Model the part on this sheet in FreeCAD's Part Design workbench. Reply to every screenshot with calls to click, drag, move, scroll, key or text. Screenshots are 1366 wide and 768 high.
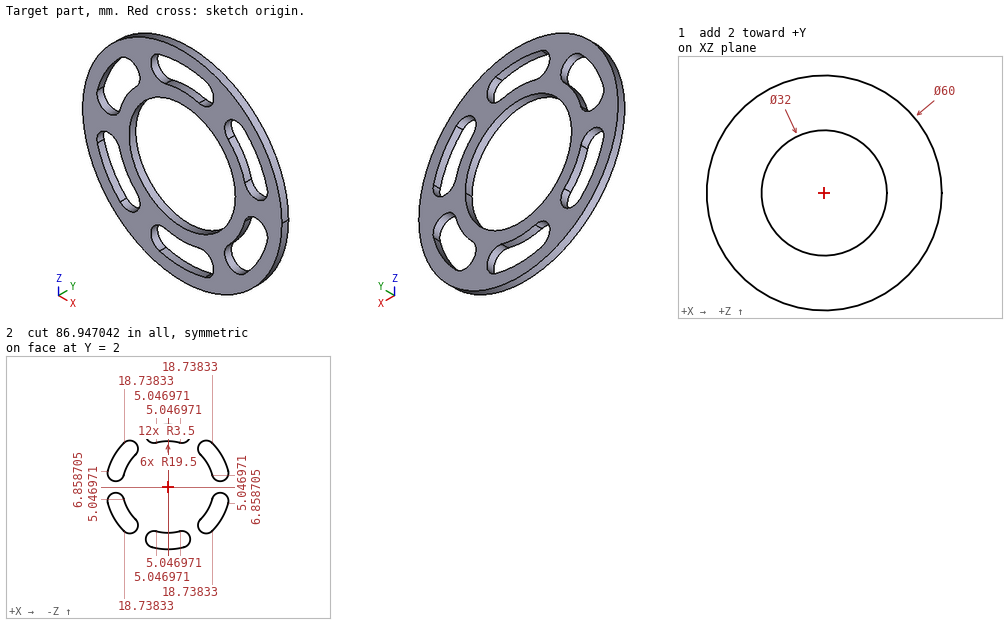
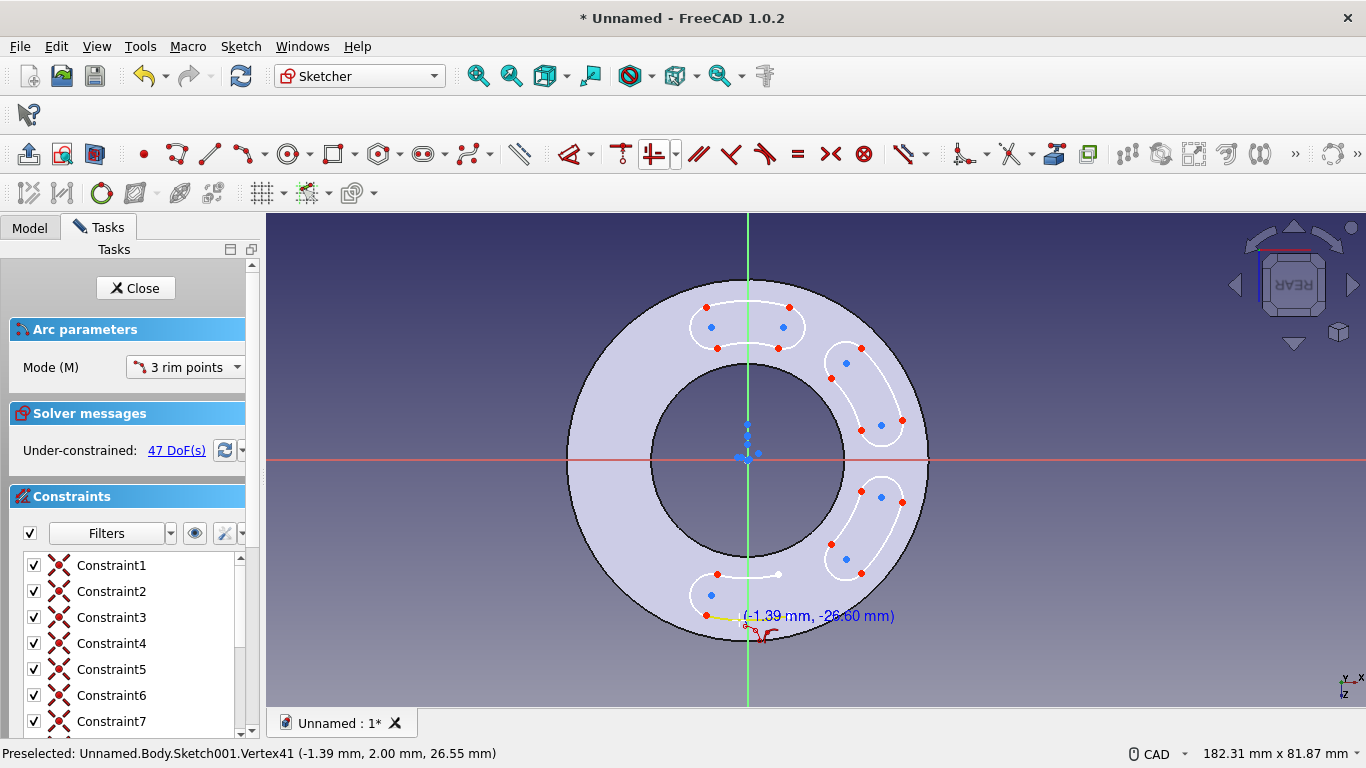
click(789, 616)
click(778, 575)
click(804, 589)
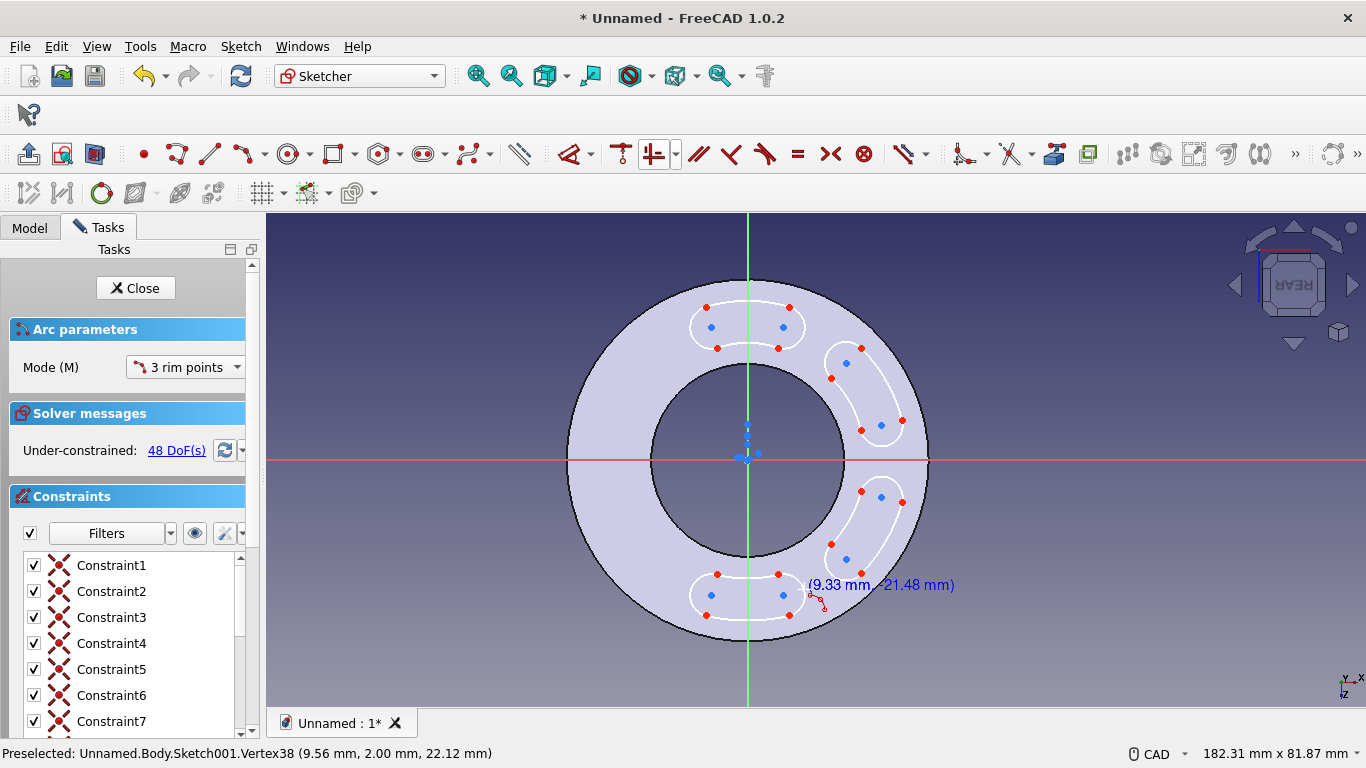
click(664, 544)
click(634, 491)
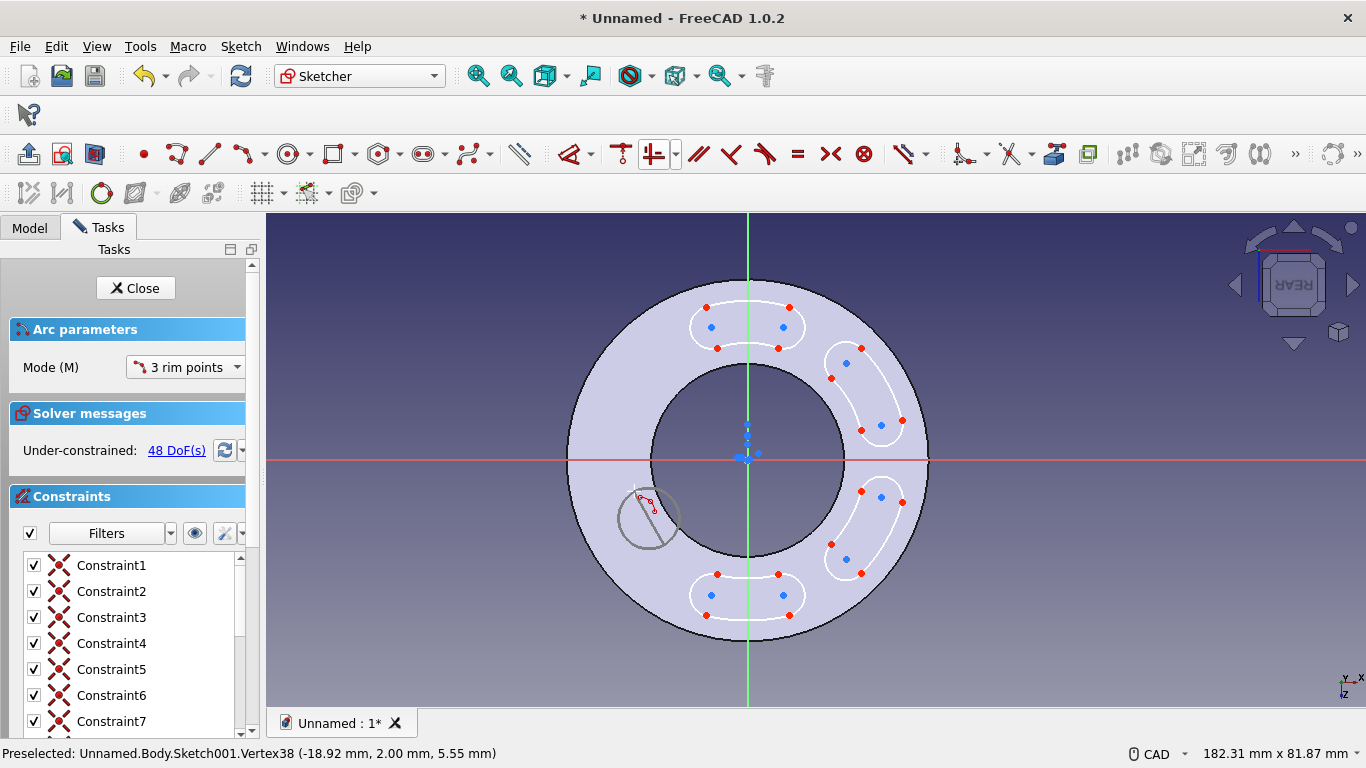
scroll(646, 519, up, 7)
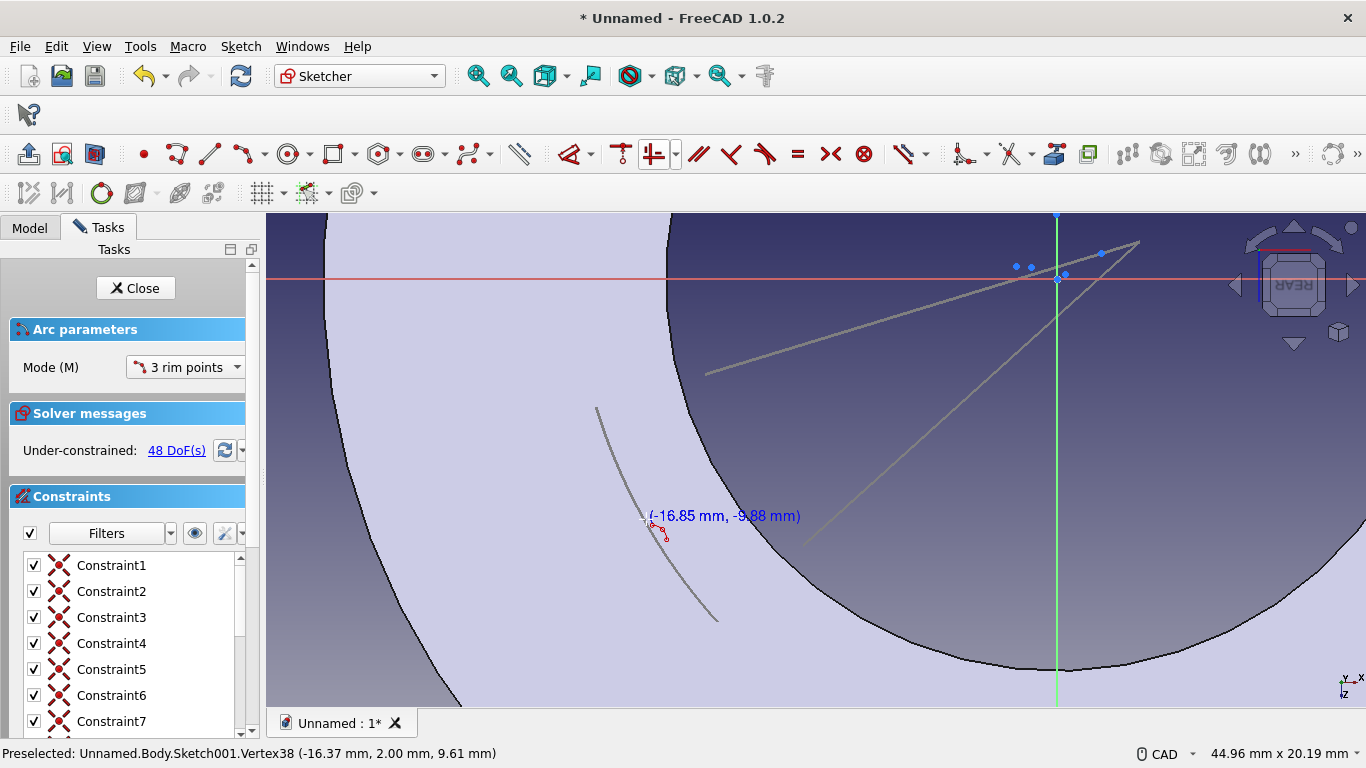
click(644, 518)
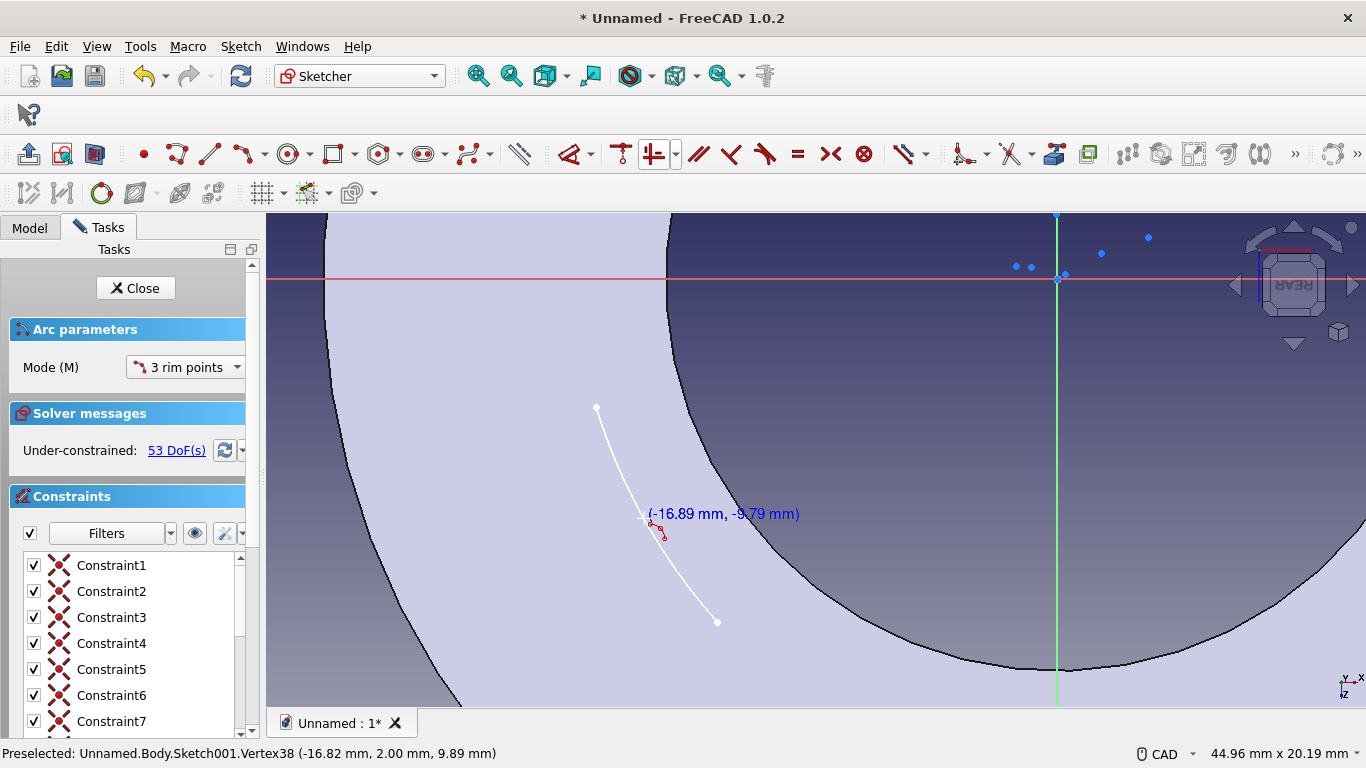
scroll(646, 519, down, 7)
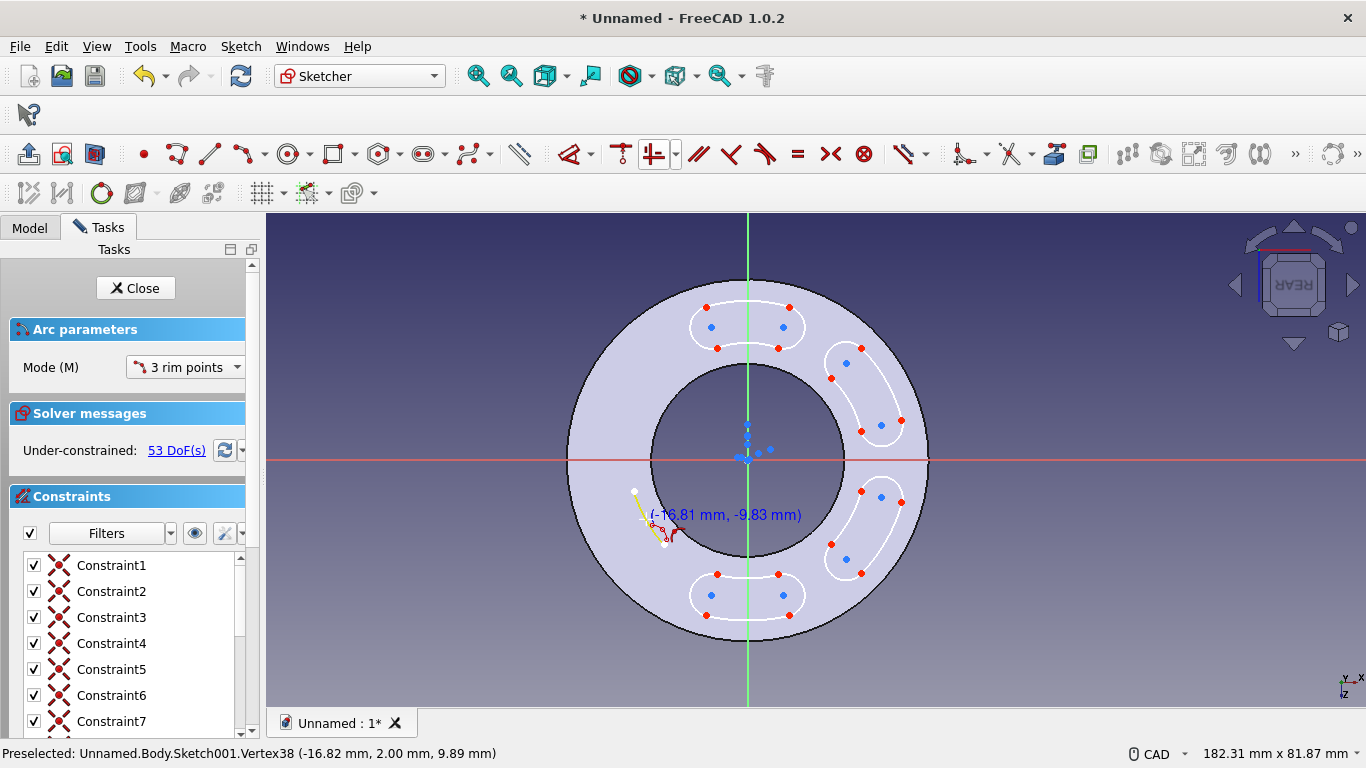
click(634, 492)
click(593, 502)
click(602, 479)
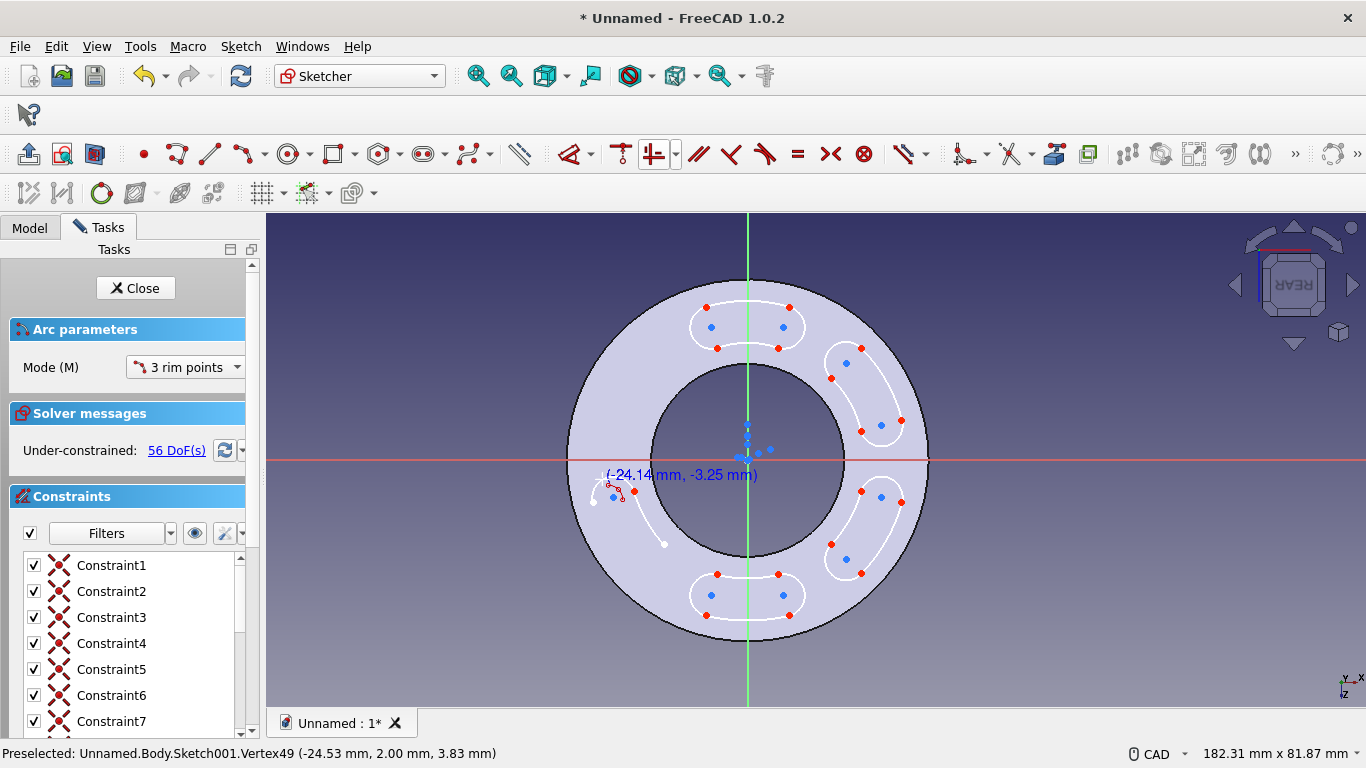
click(593, 503)
click(635, 573)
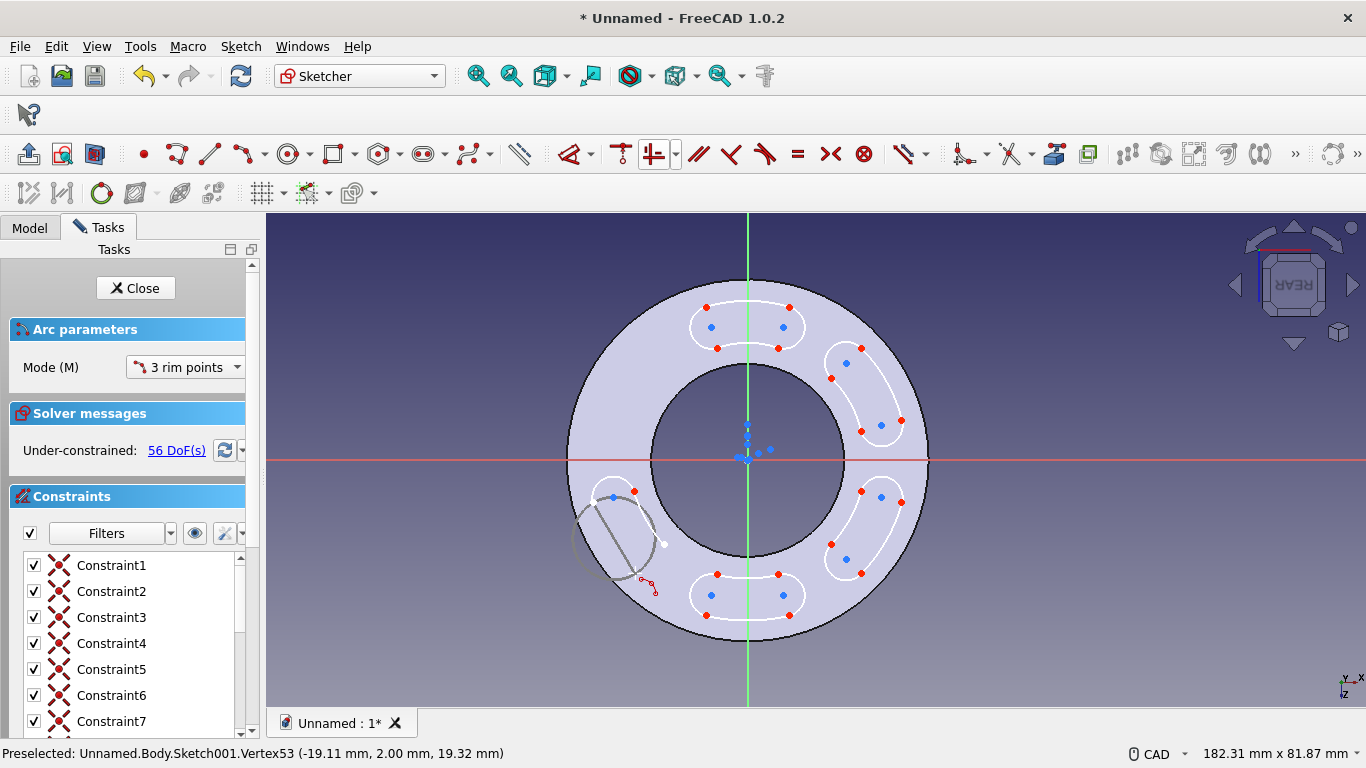
scroll(609, 540, up, 6)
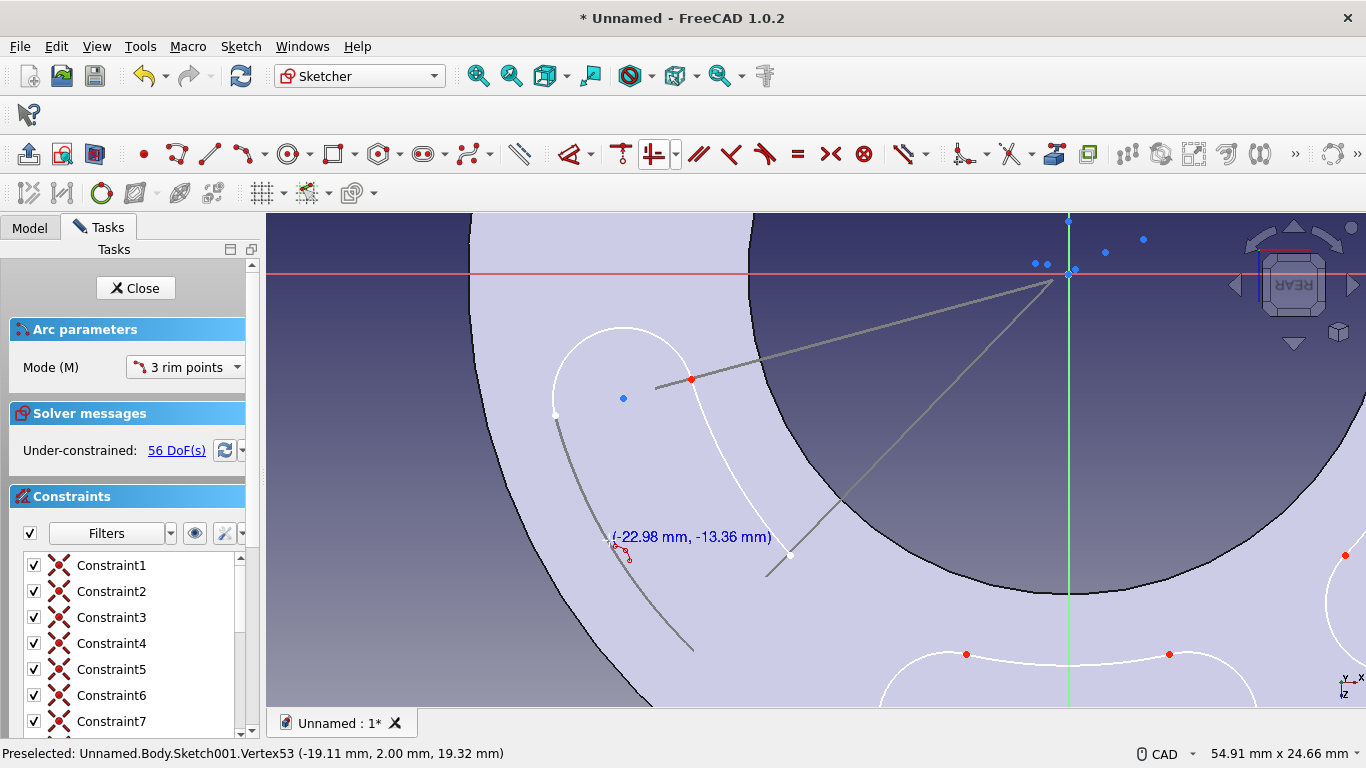
click(609, 540)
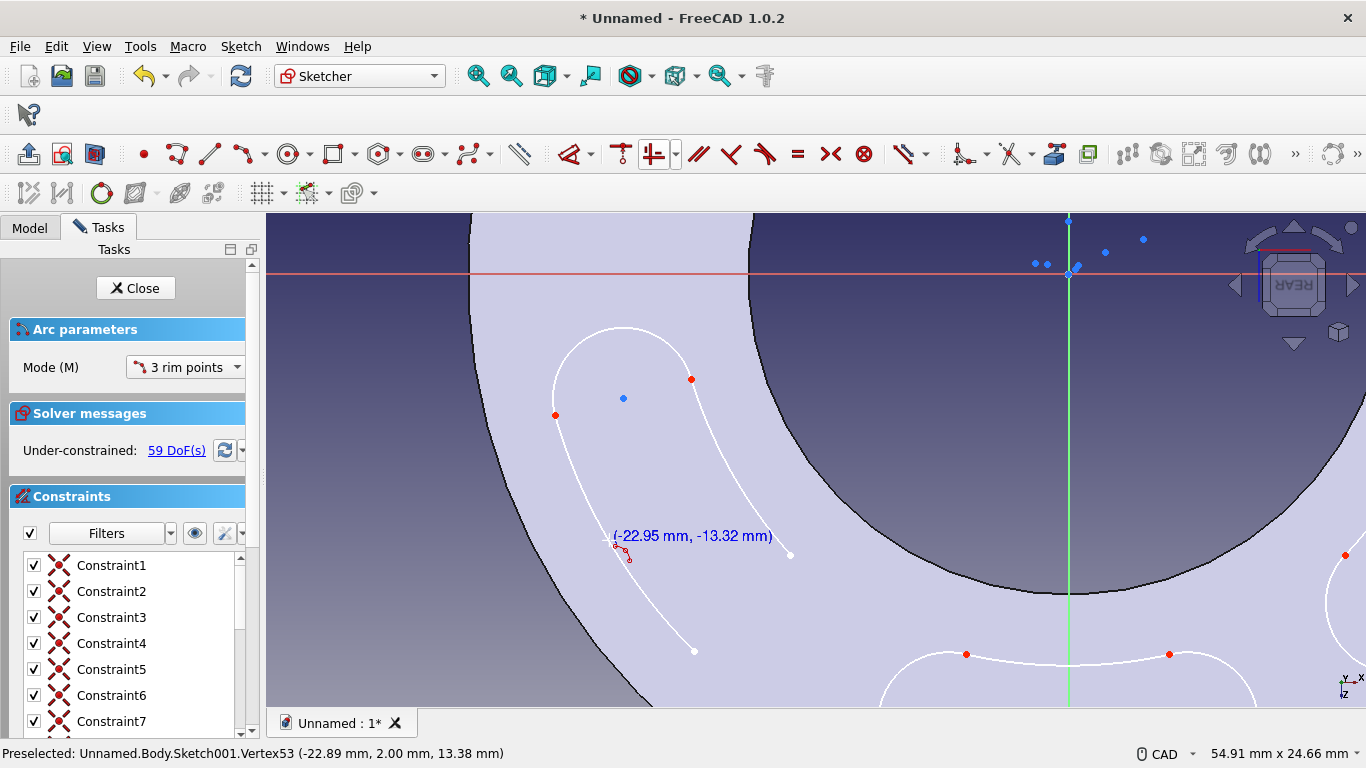
scroll(609, 540, down, 6)